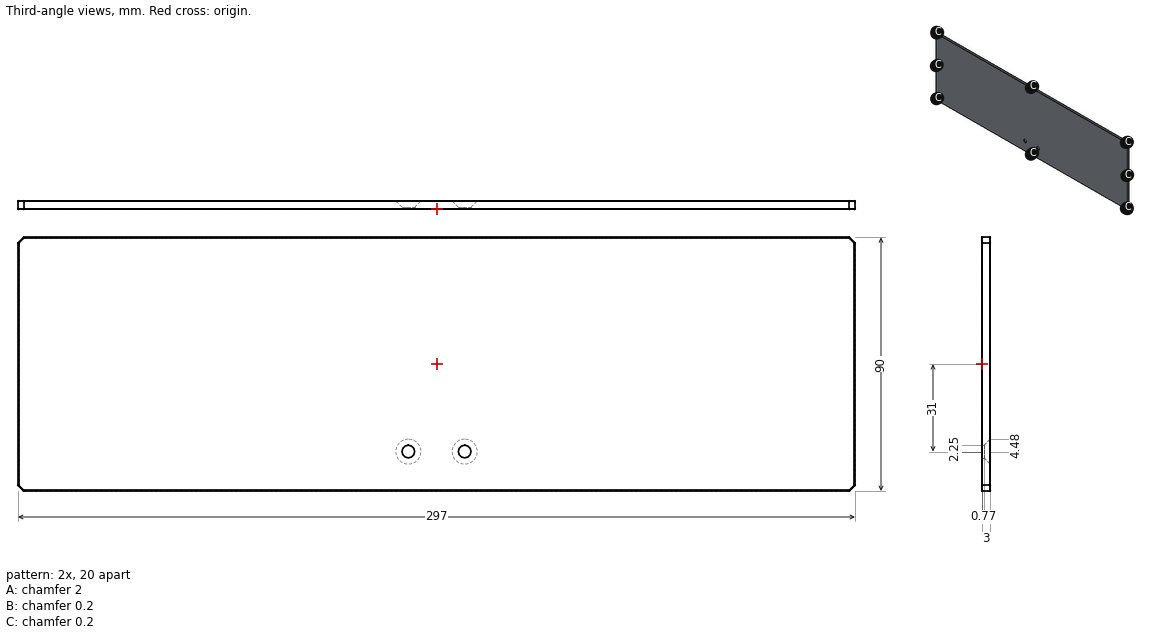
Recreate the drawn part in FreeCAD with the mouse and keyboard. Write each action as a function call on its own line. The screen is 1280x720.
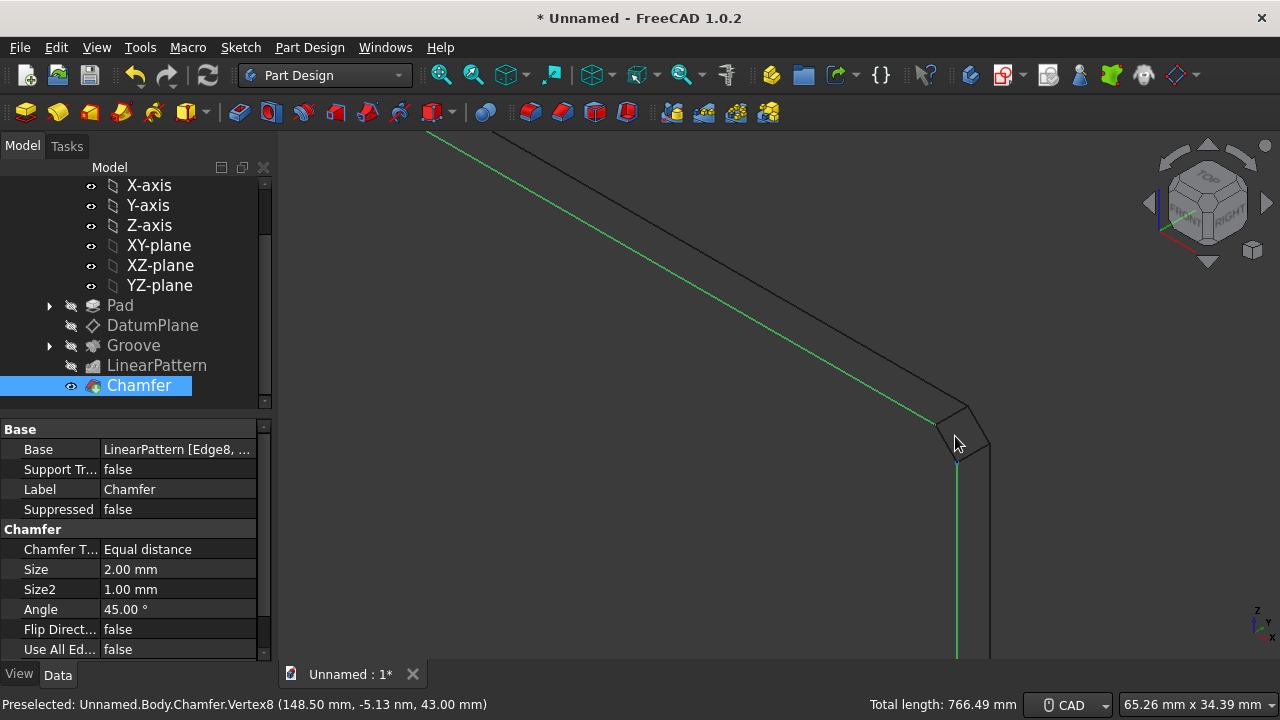
click(946, 443, ctrl)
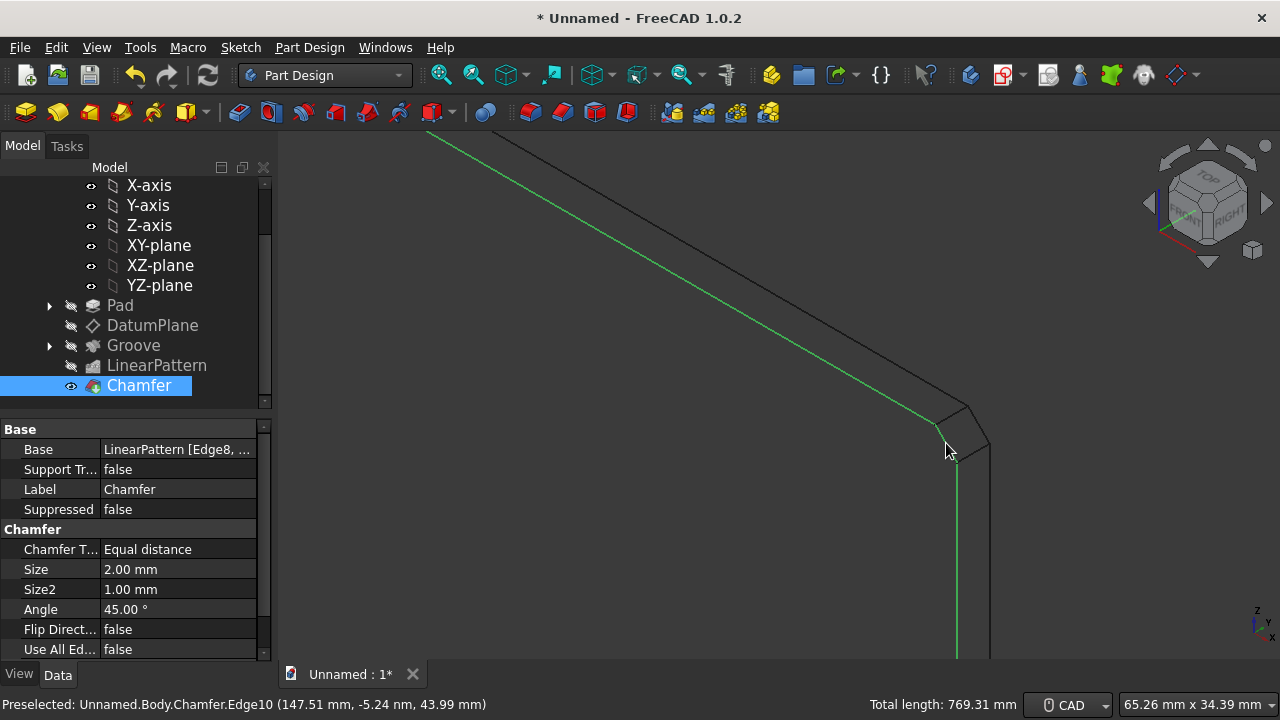
key(v)
key(1)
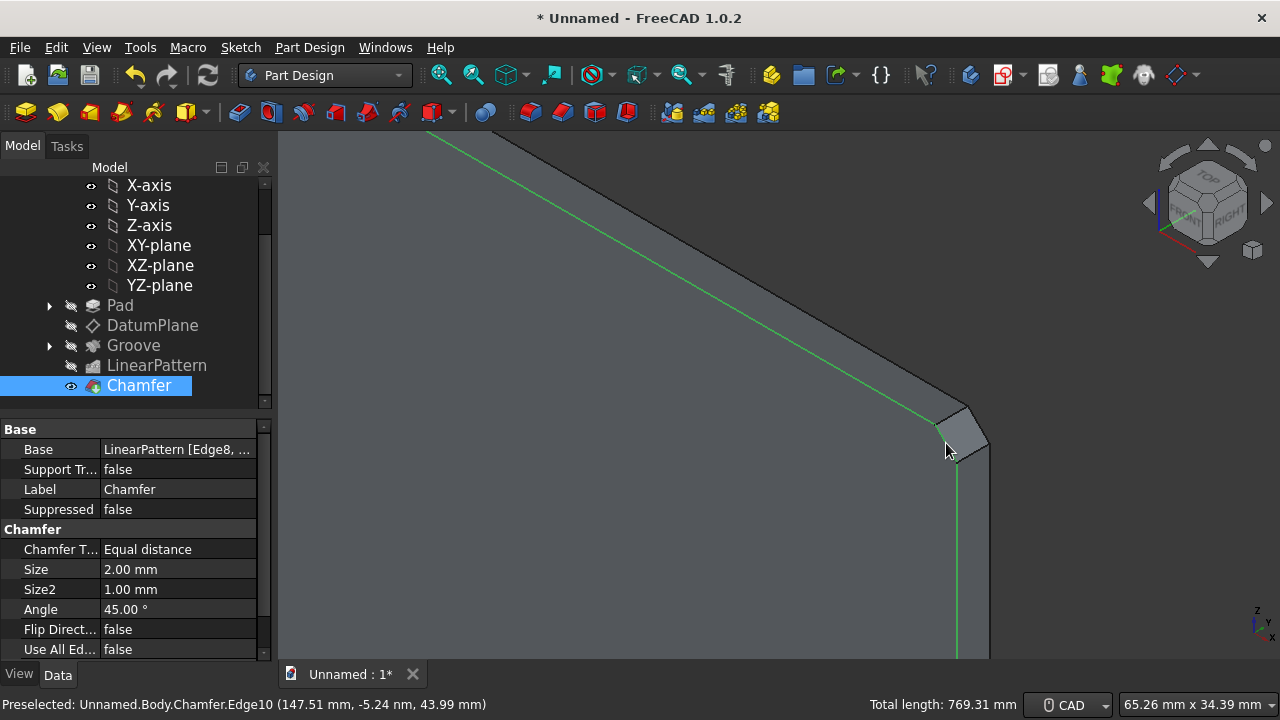
click(564, 112)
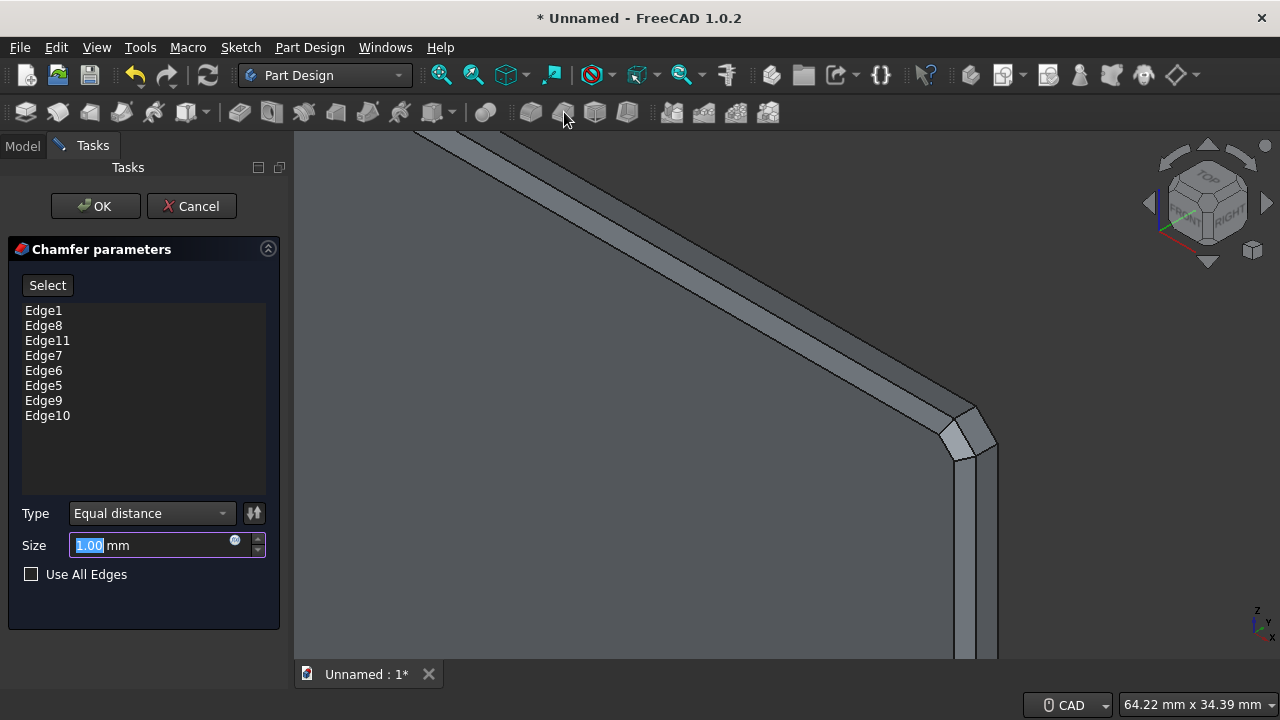
text(0.2)
key(Tab)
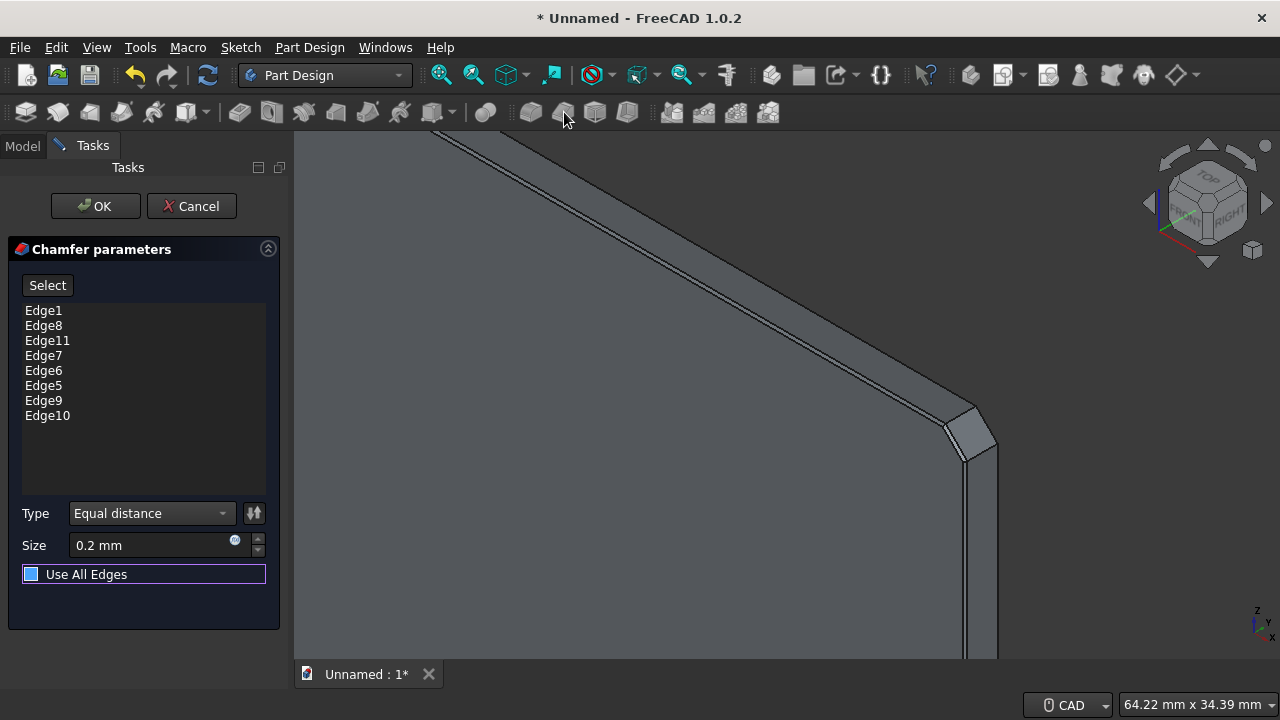
click(96, 206)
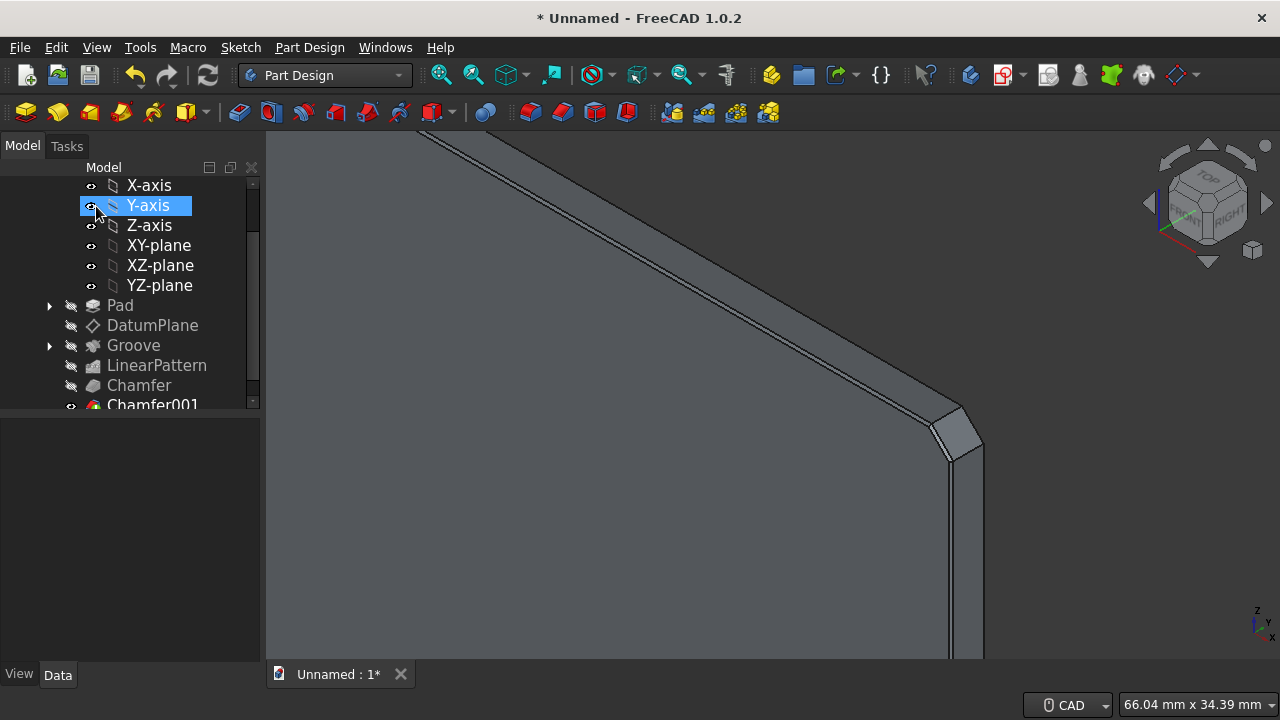
key(v)
key(f)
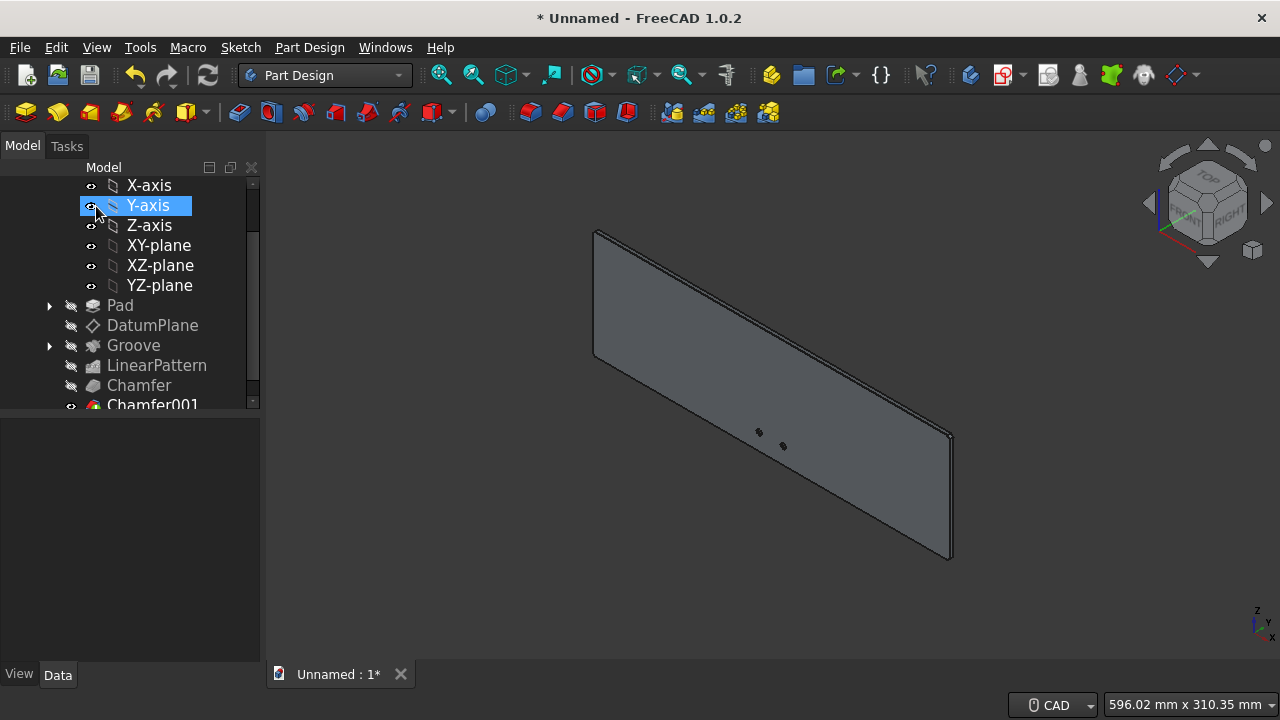
key(2)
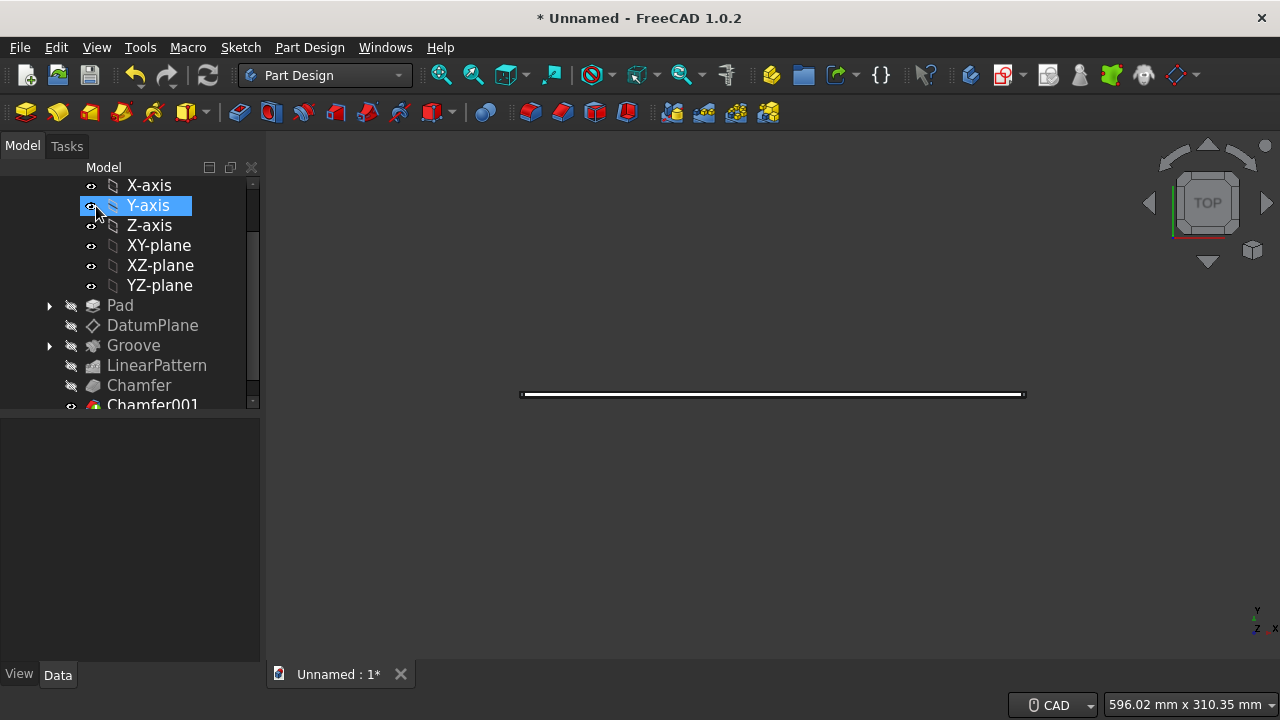
click(773, 391)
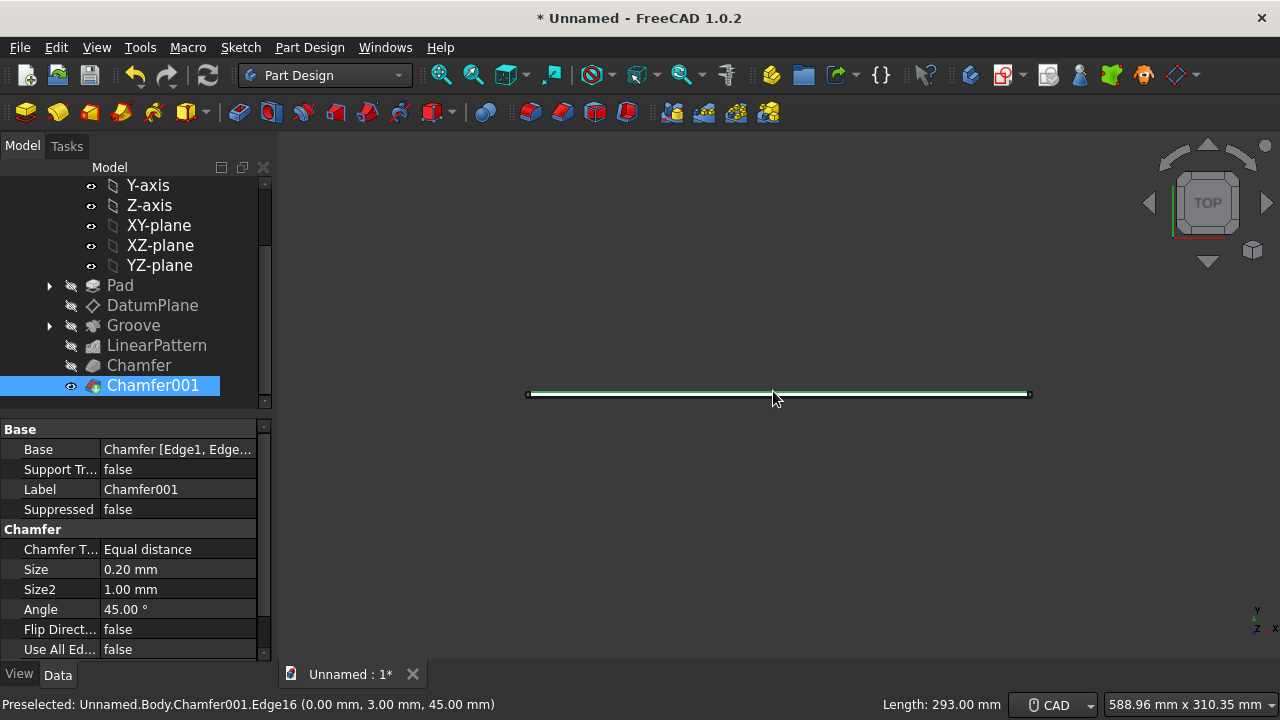
key(0)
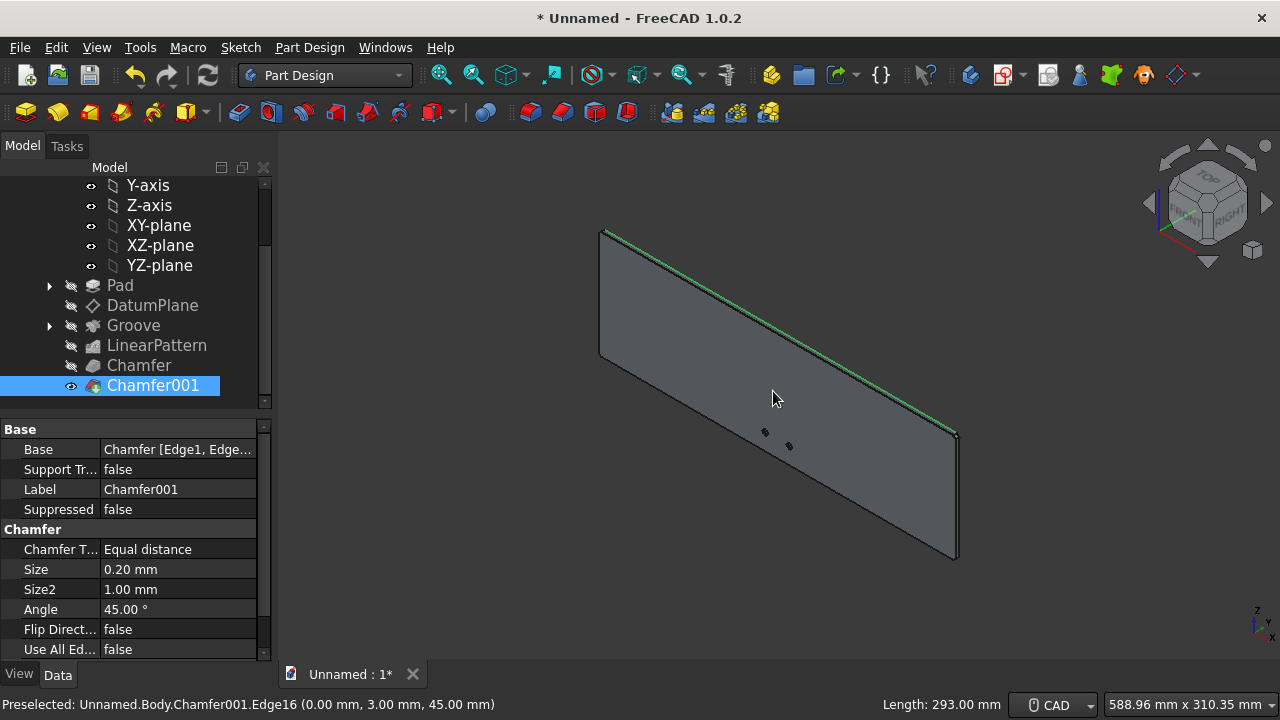
key(1)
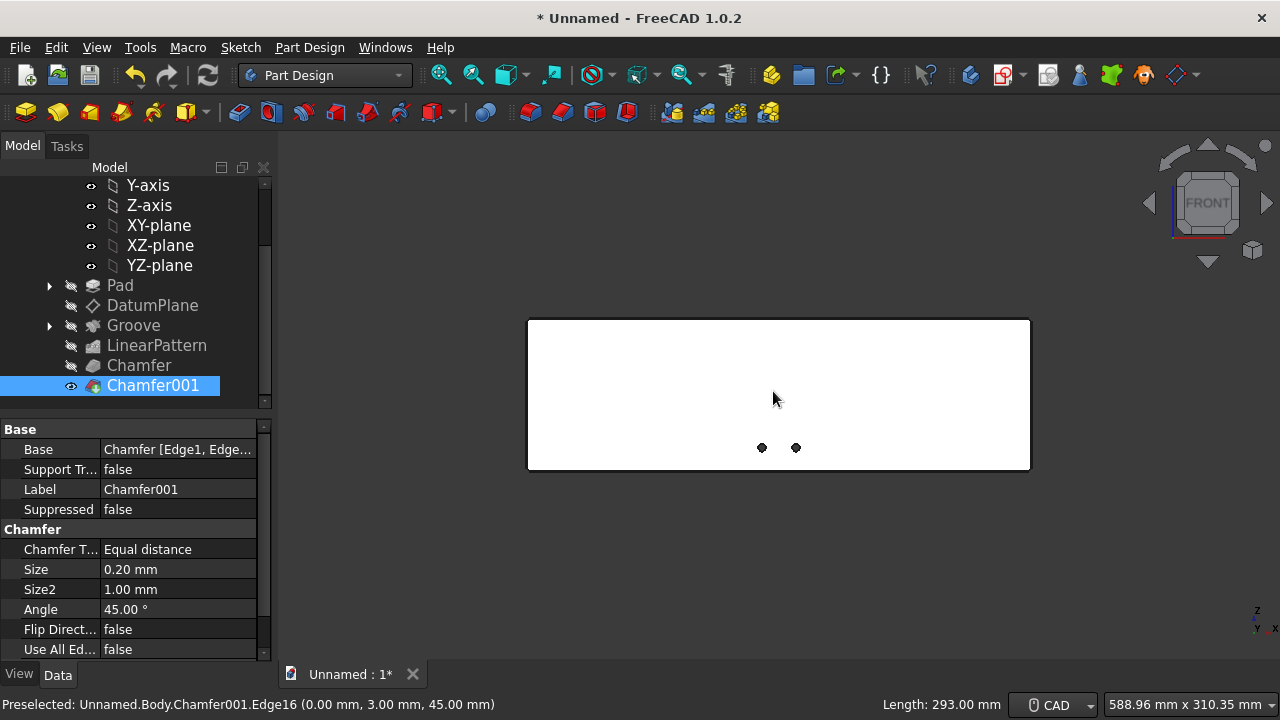
key(3)